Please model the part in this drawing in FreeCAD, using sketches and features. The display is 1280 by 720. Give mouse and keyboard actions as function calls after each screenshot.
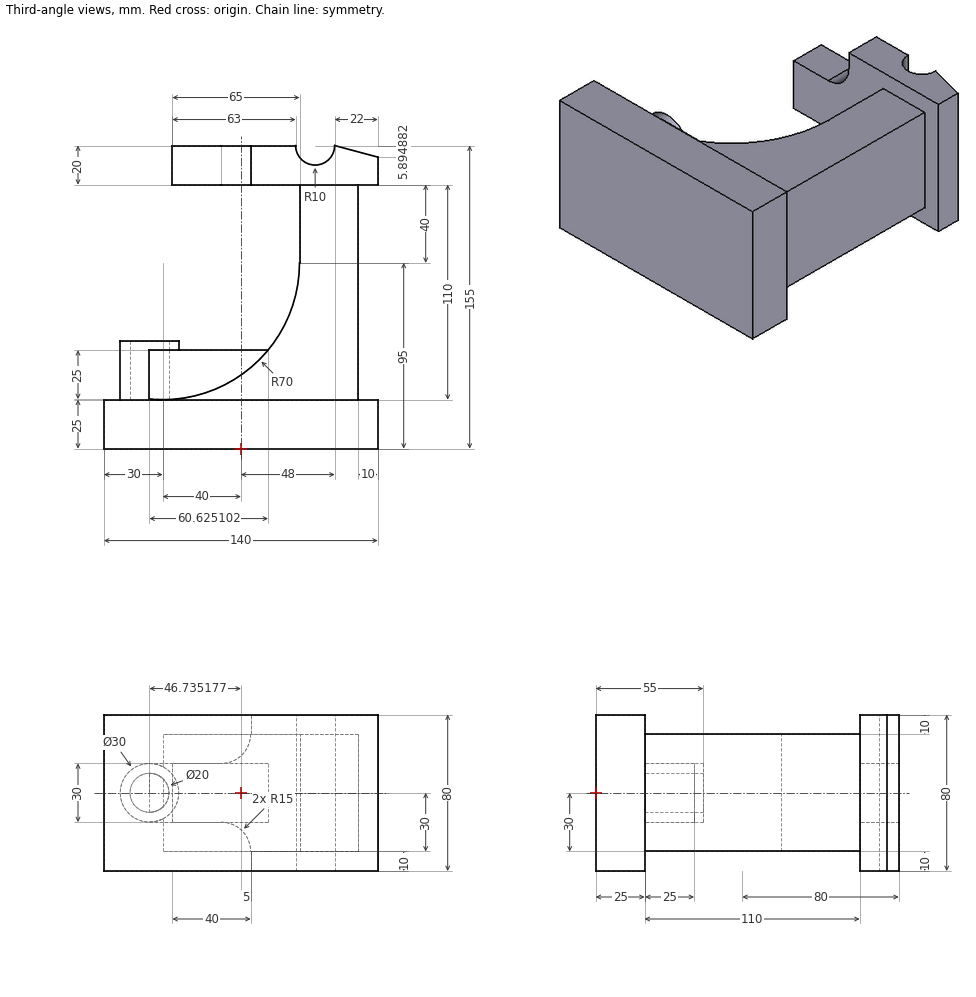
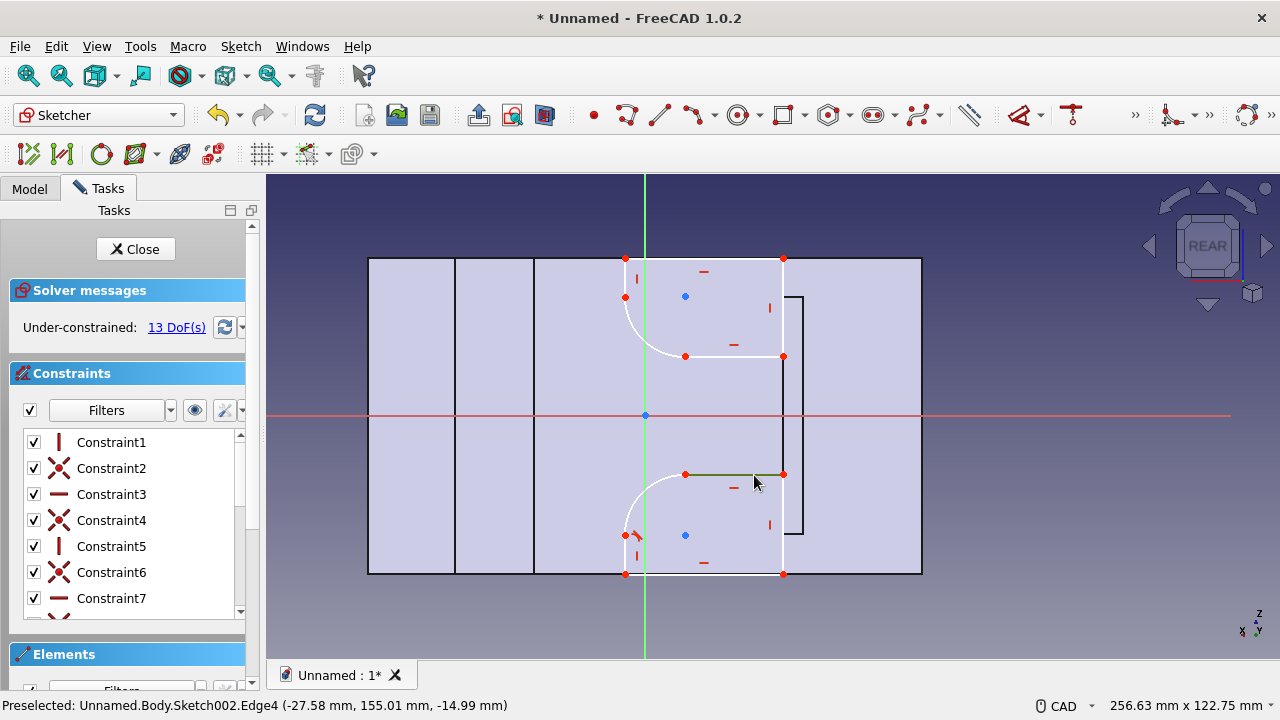
click(658, 482)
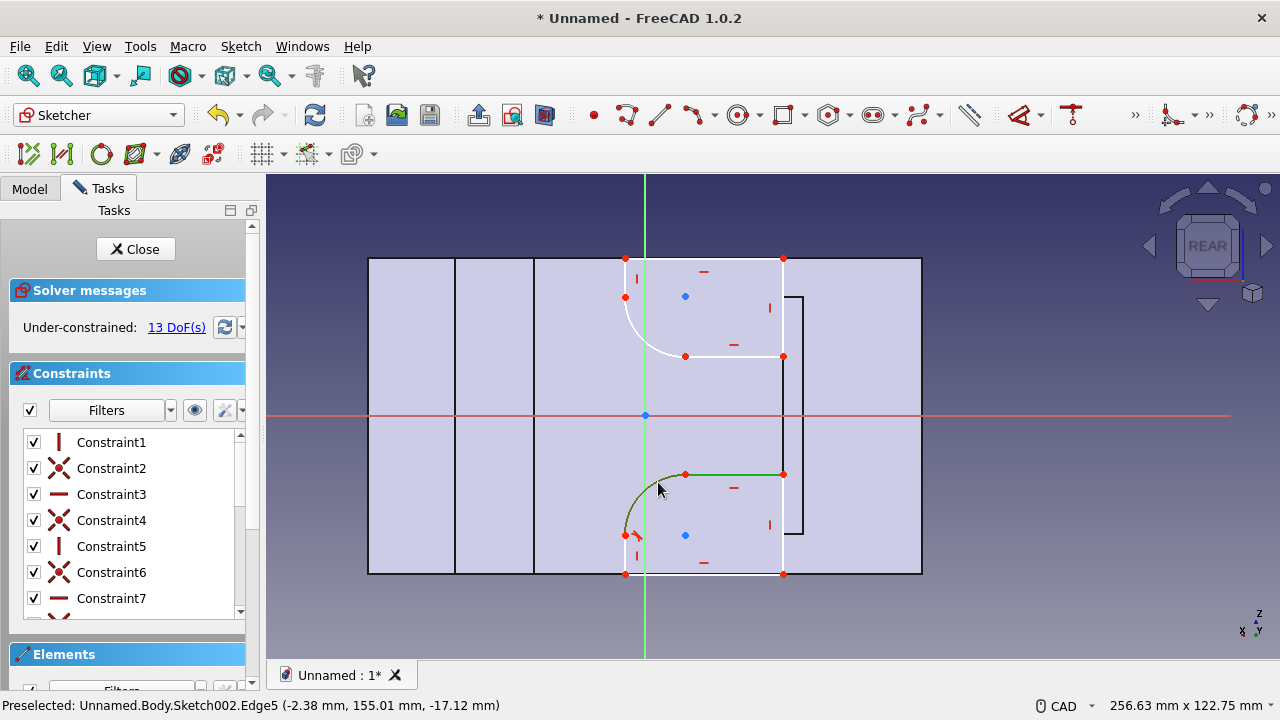
key(t)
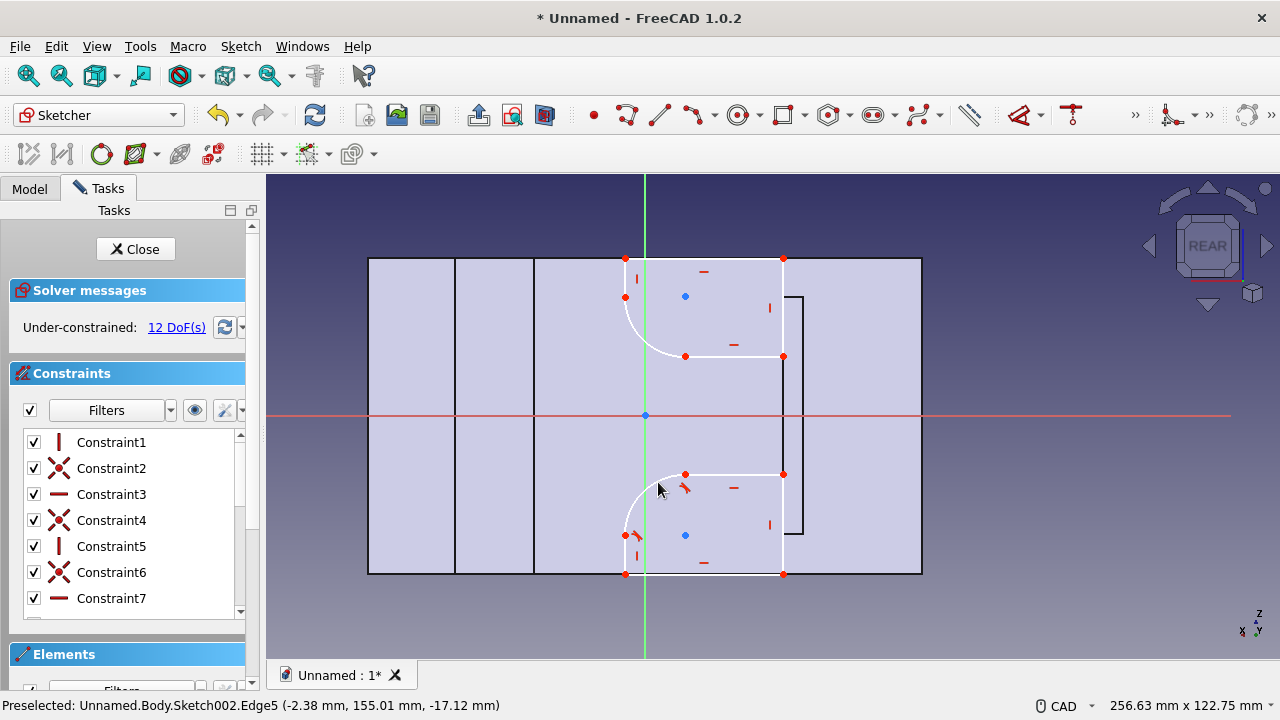
click(714, 357)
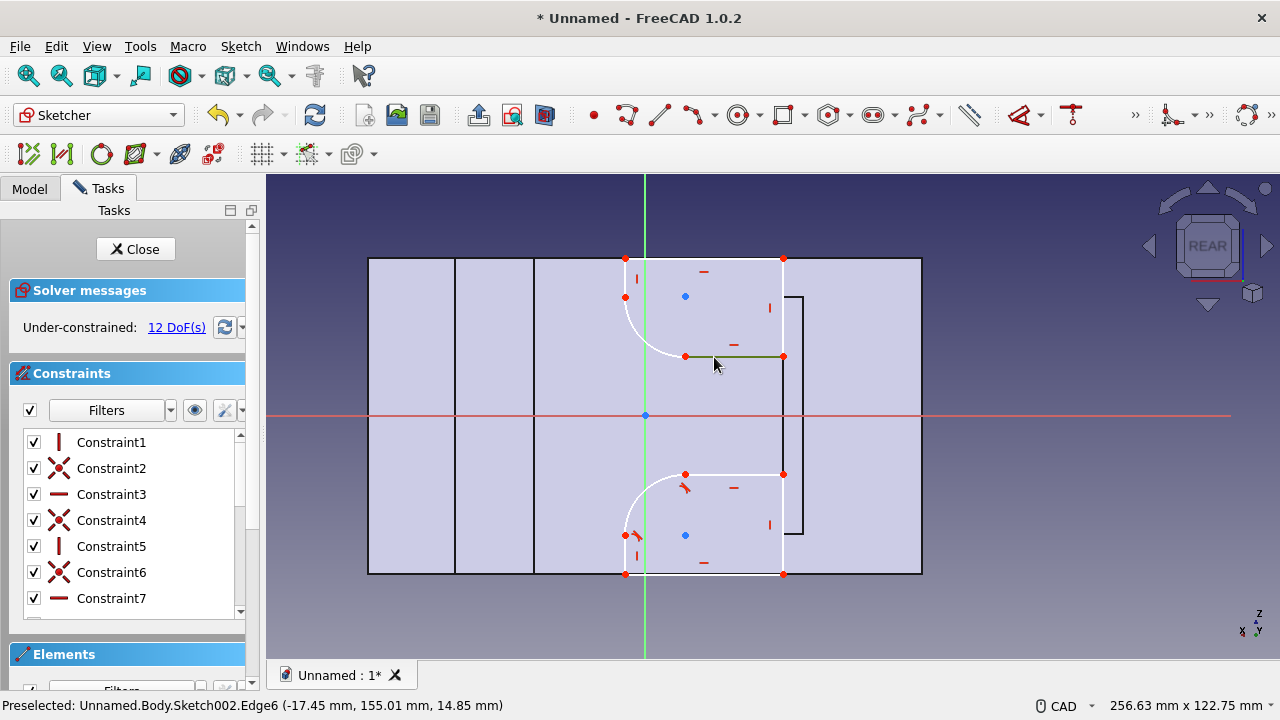
click(632, 325)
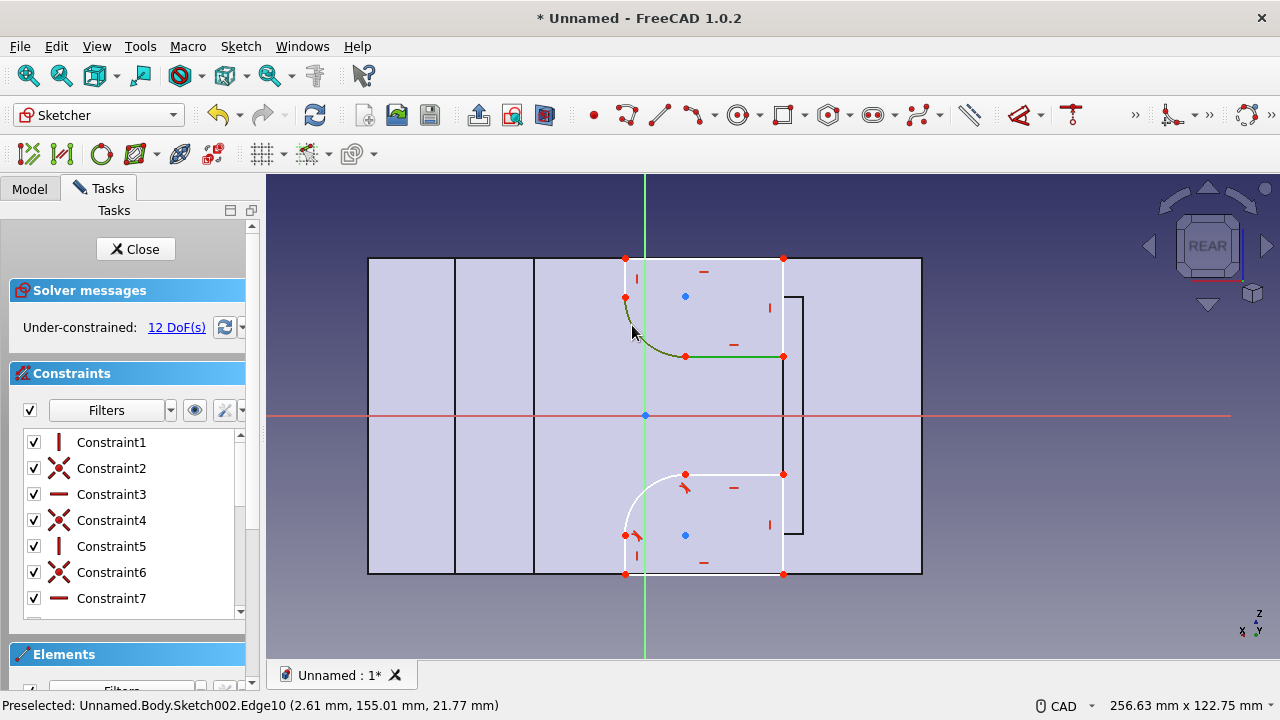
key(t)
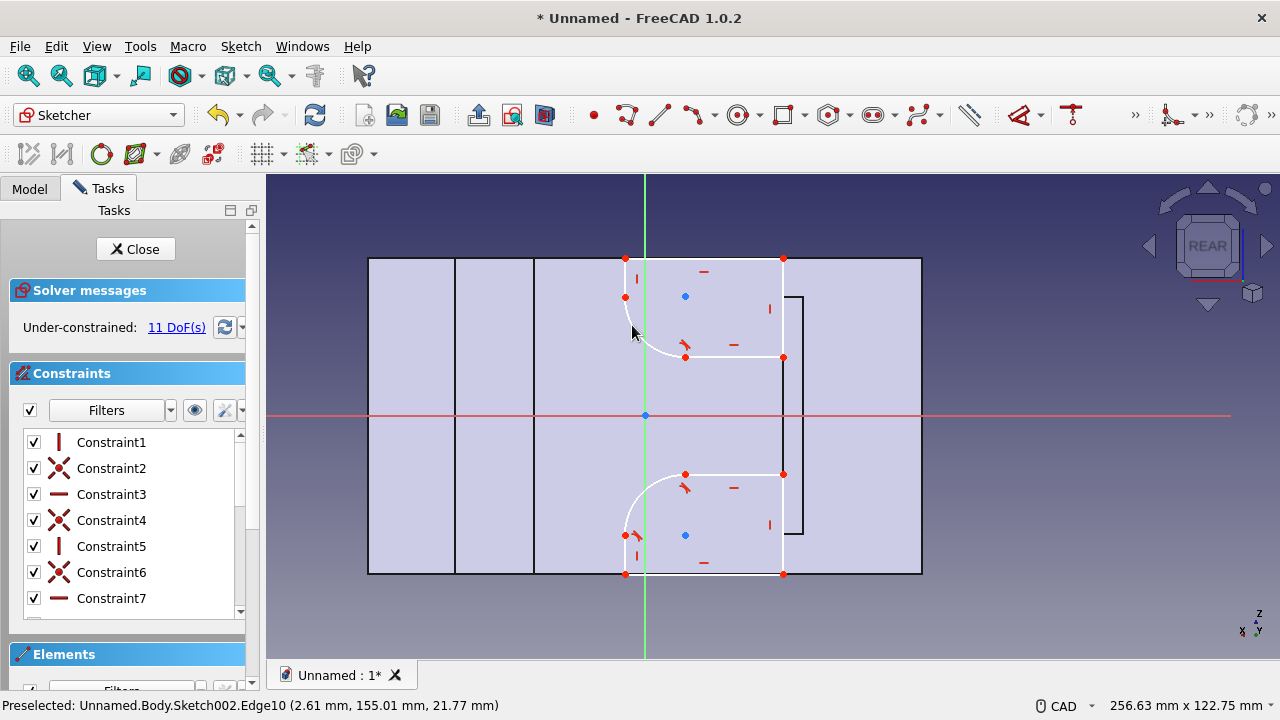
click(625, 271)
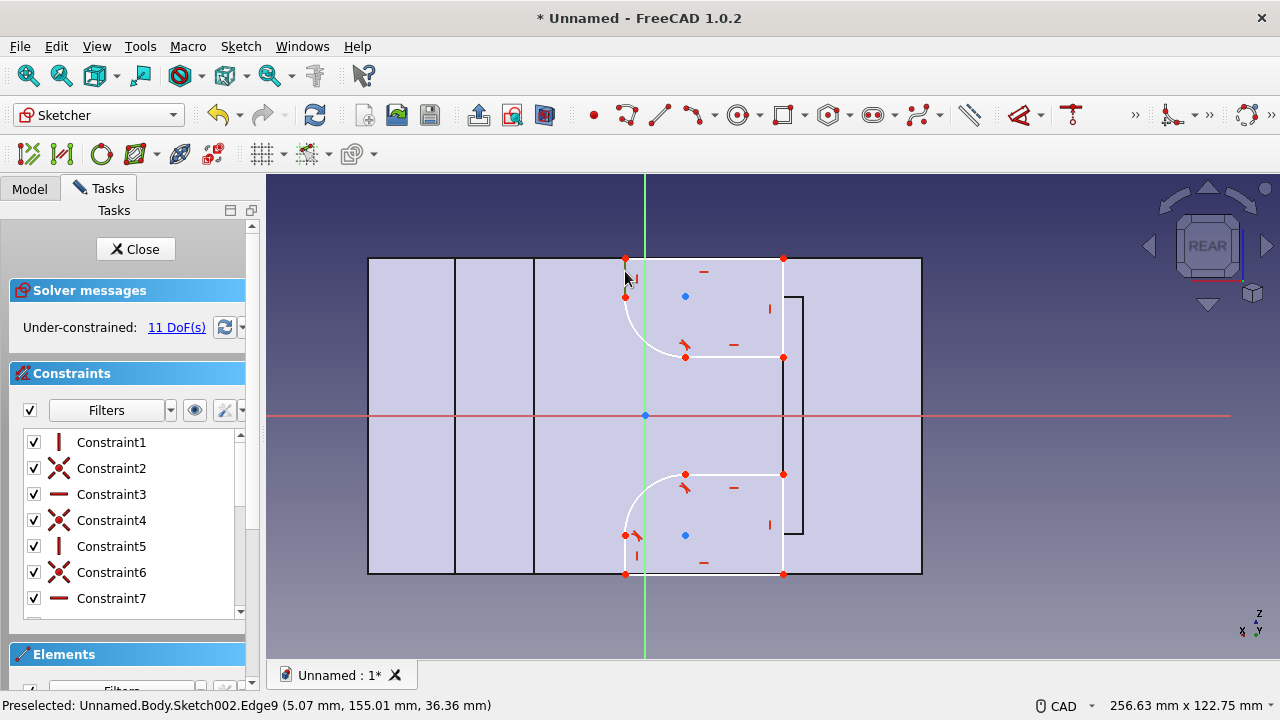
click(632, 325)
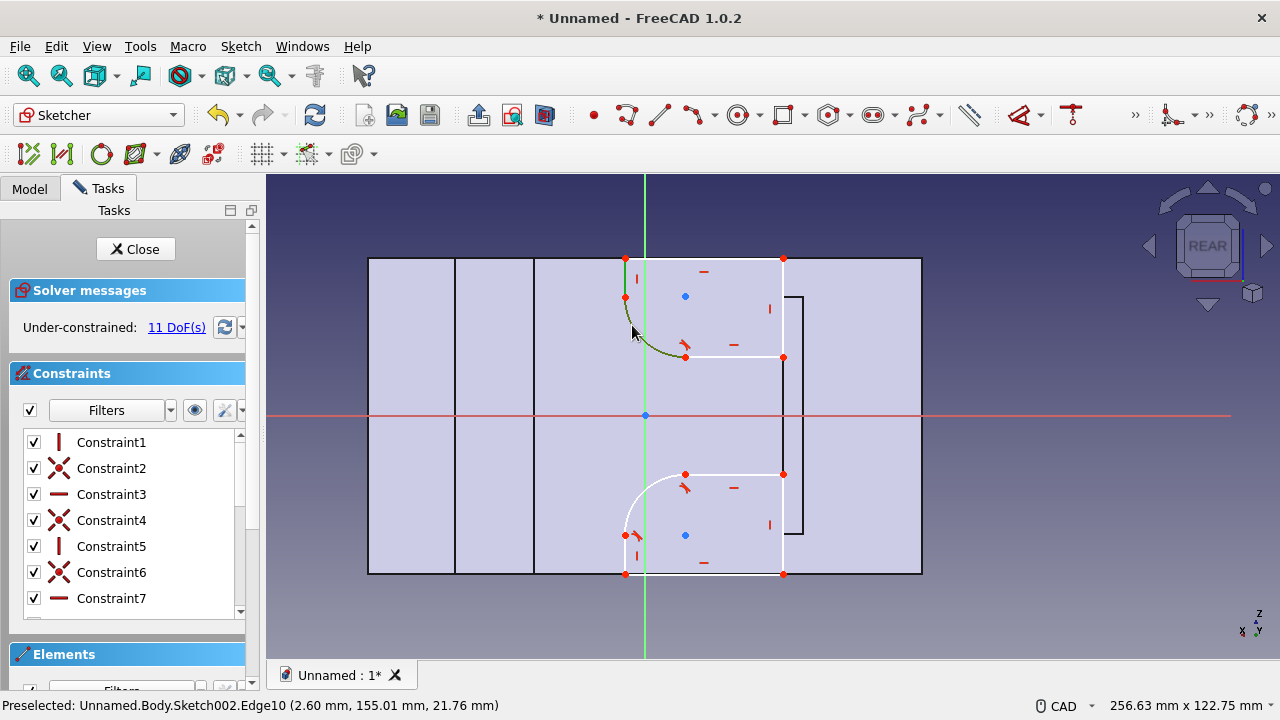
key(t)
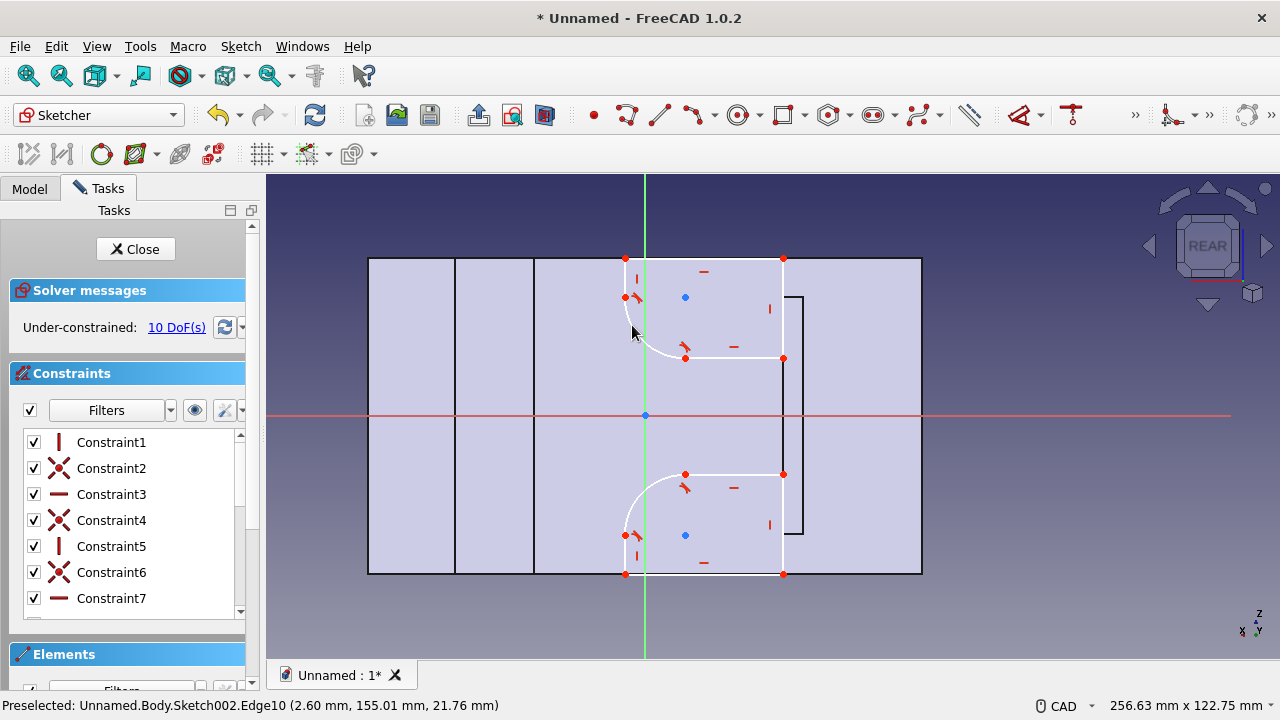
click(658, 481)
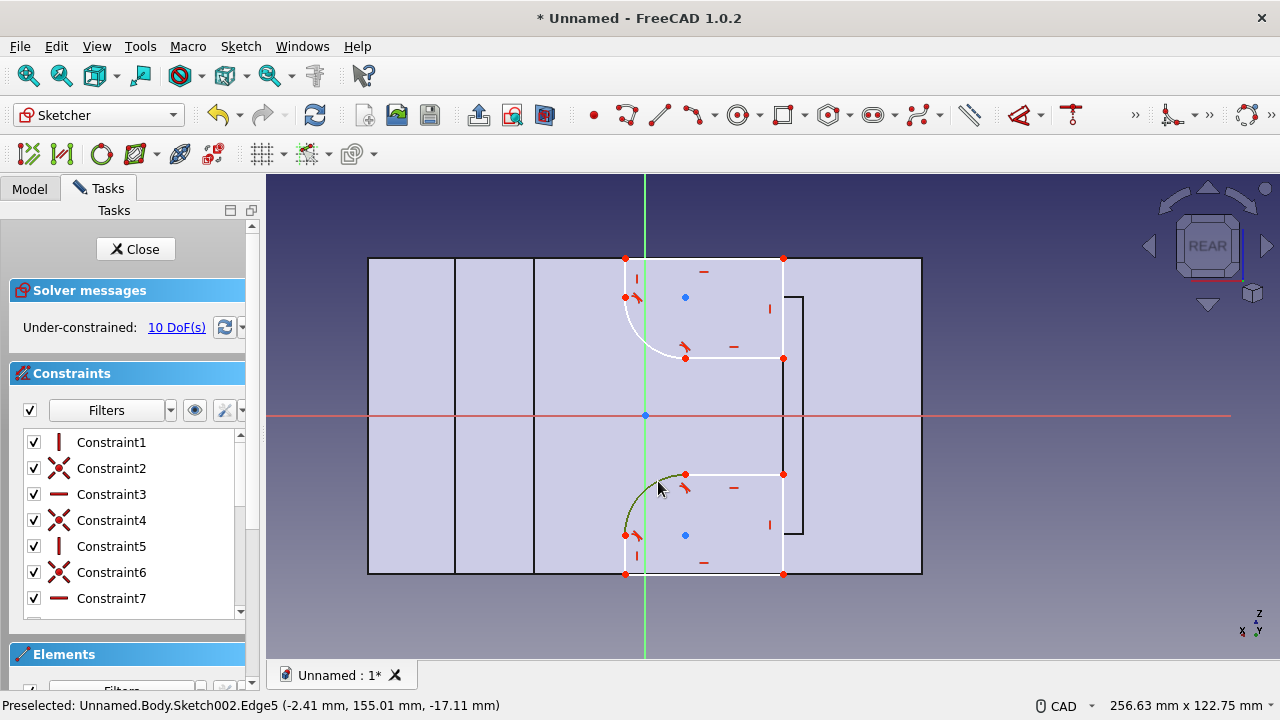
click(632, 325)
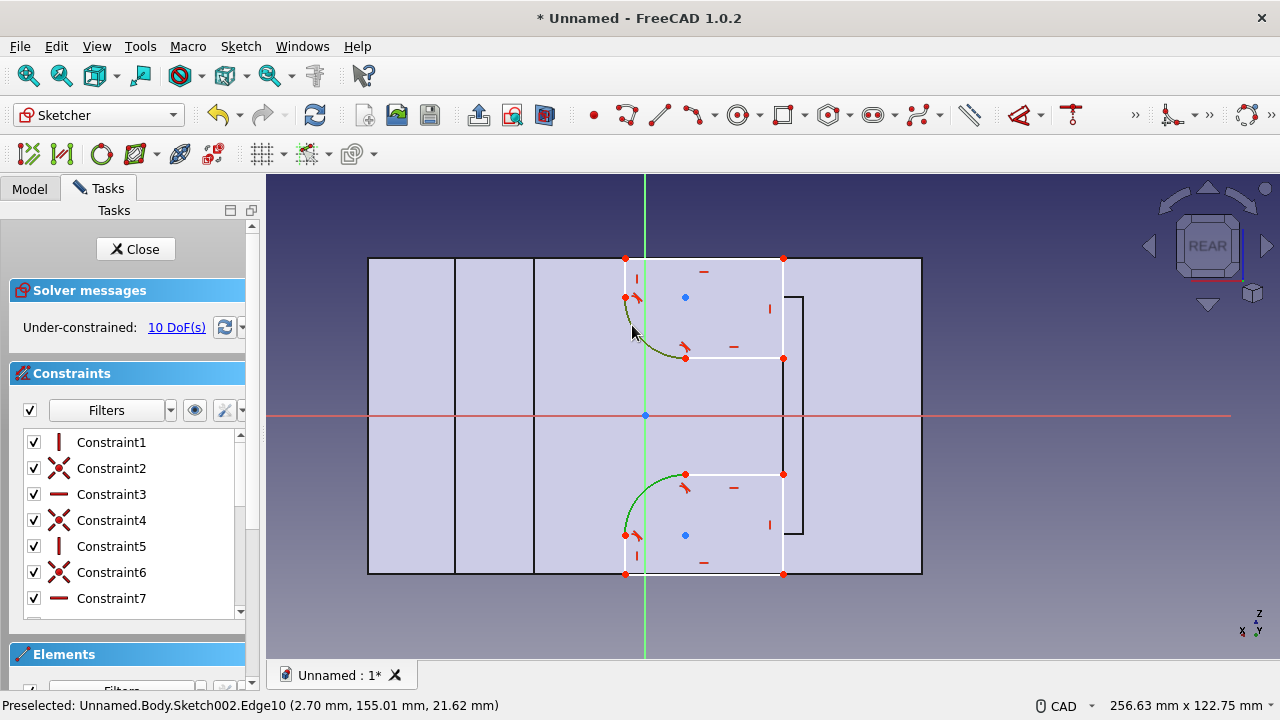
key(e)